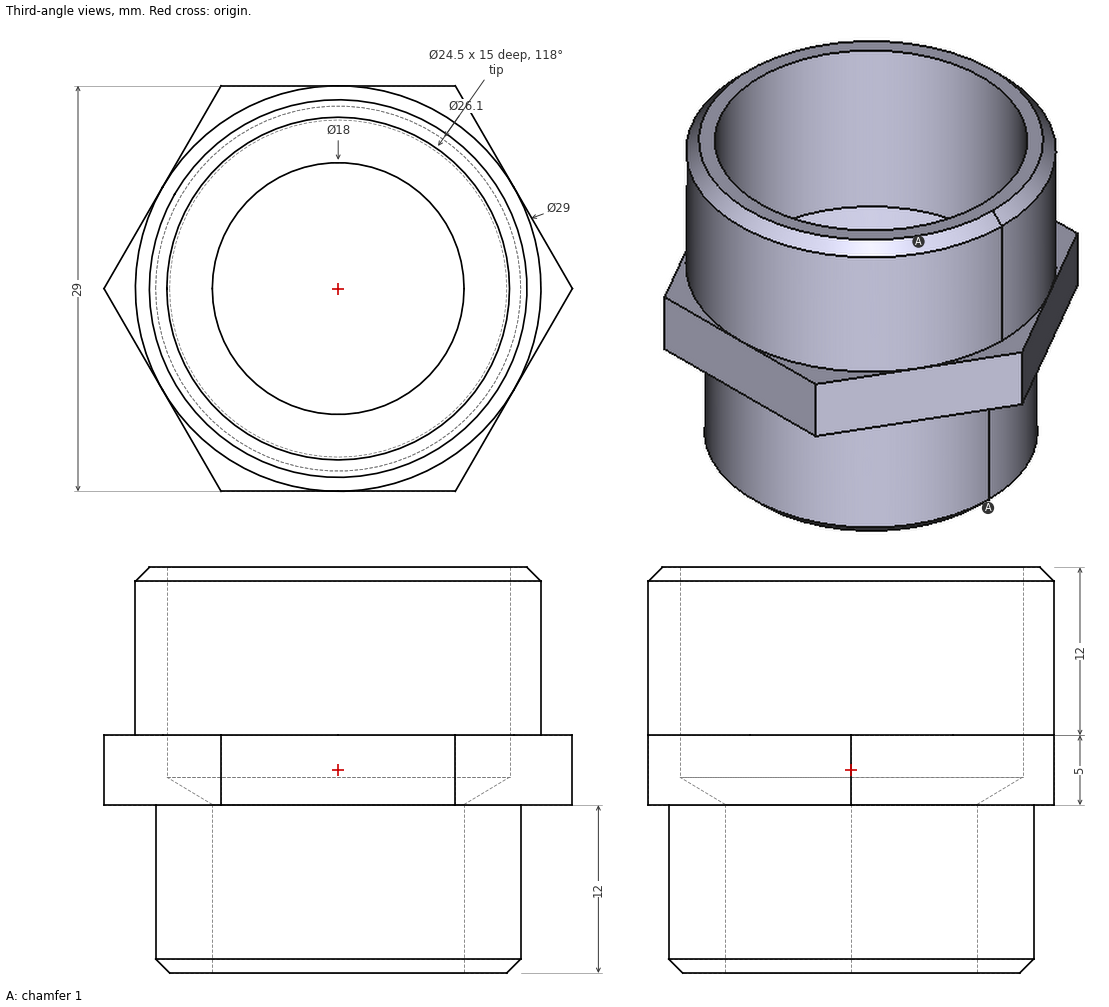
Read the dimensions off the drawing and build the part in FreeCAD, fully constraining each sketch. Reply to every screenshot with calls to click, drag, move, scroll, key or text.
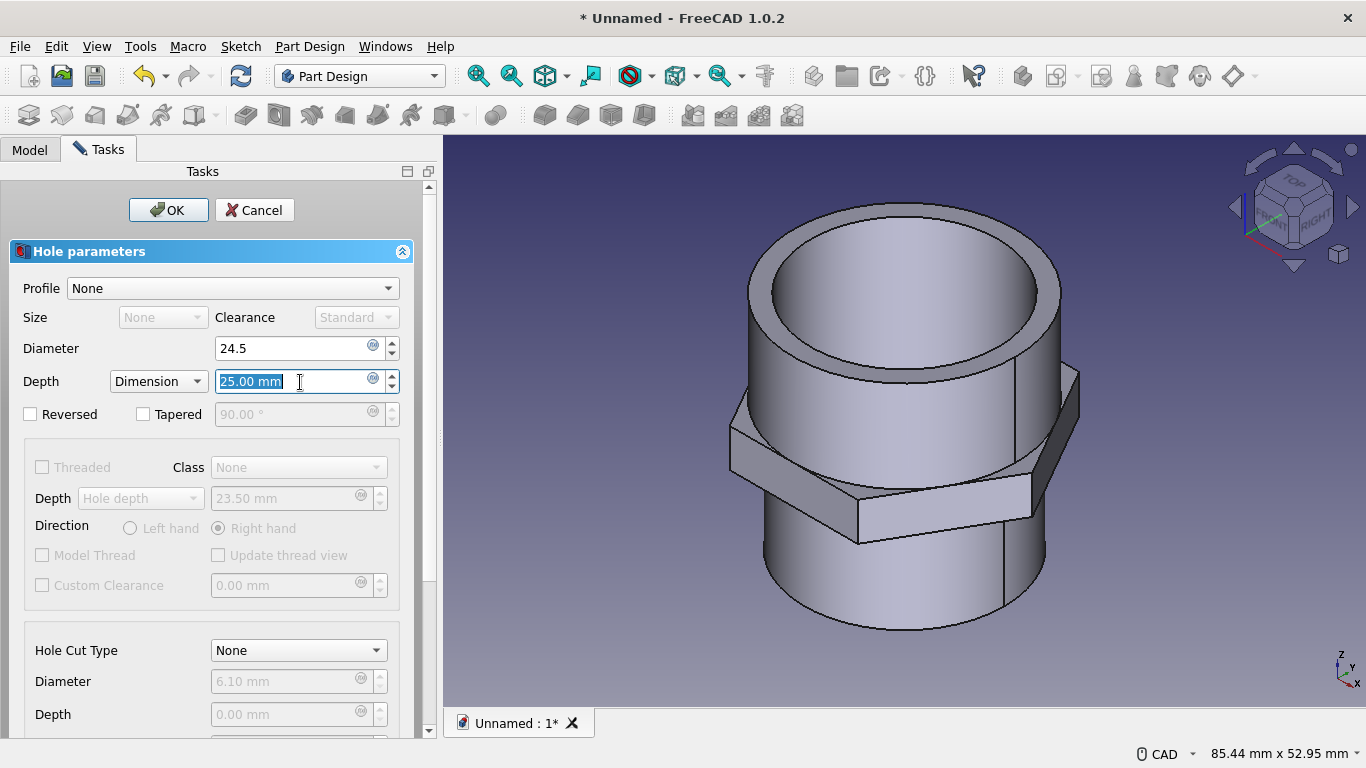
text(15)
key(Tab)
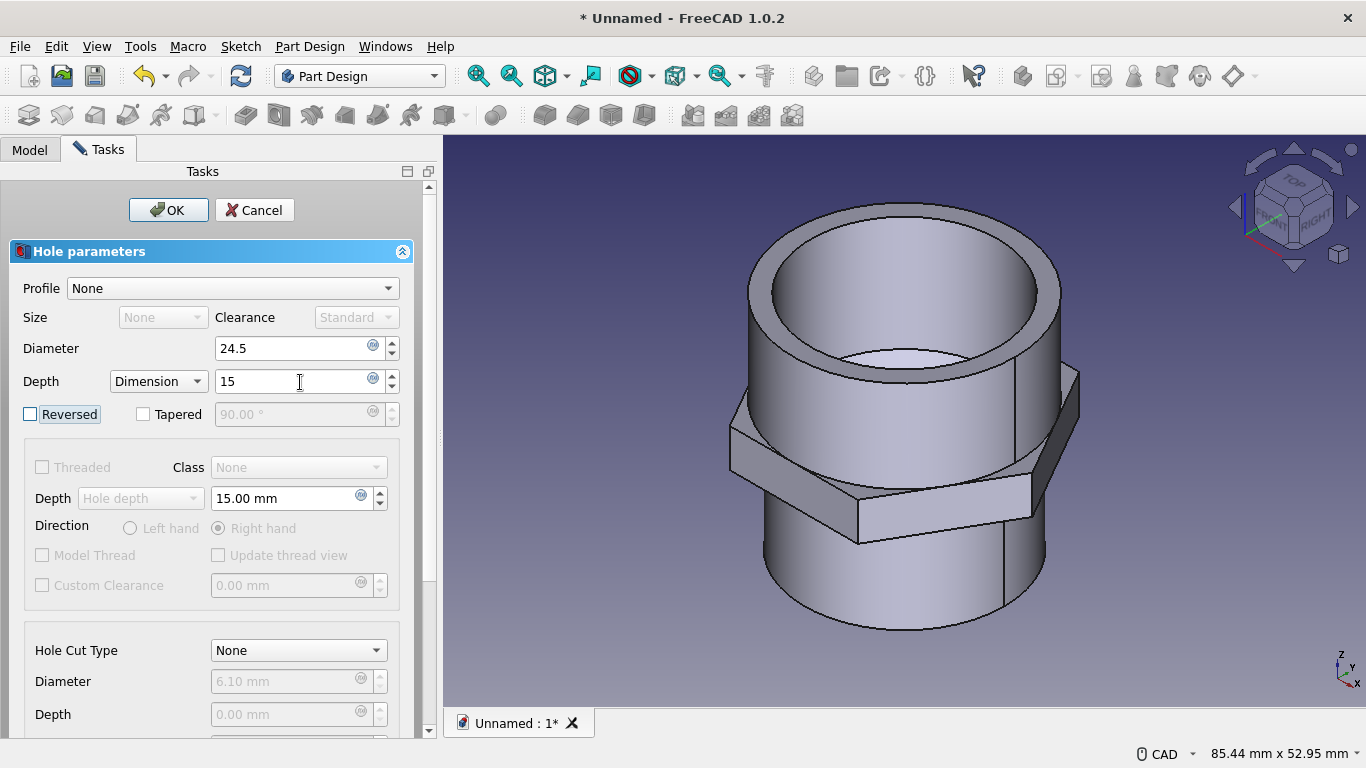
click(169, 210)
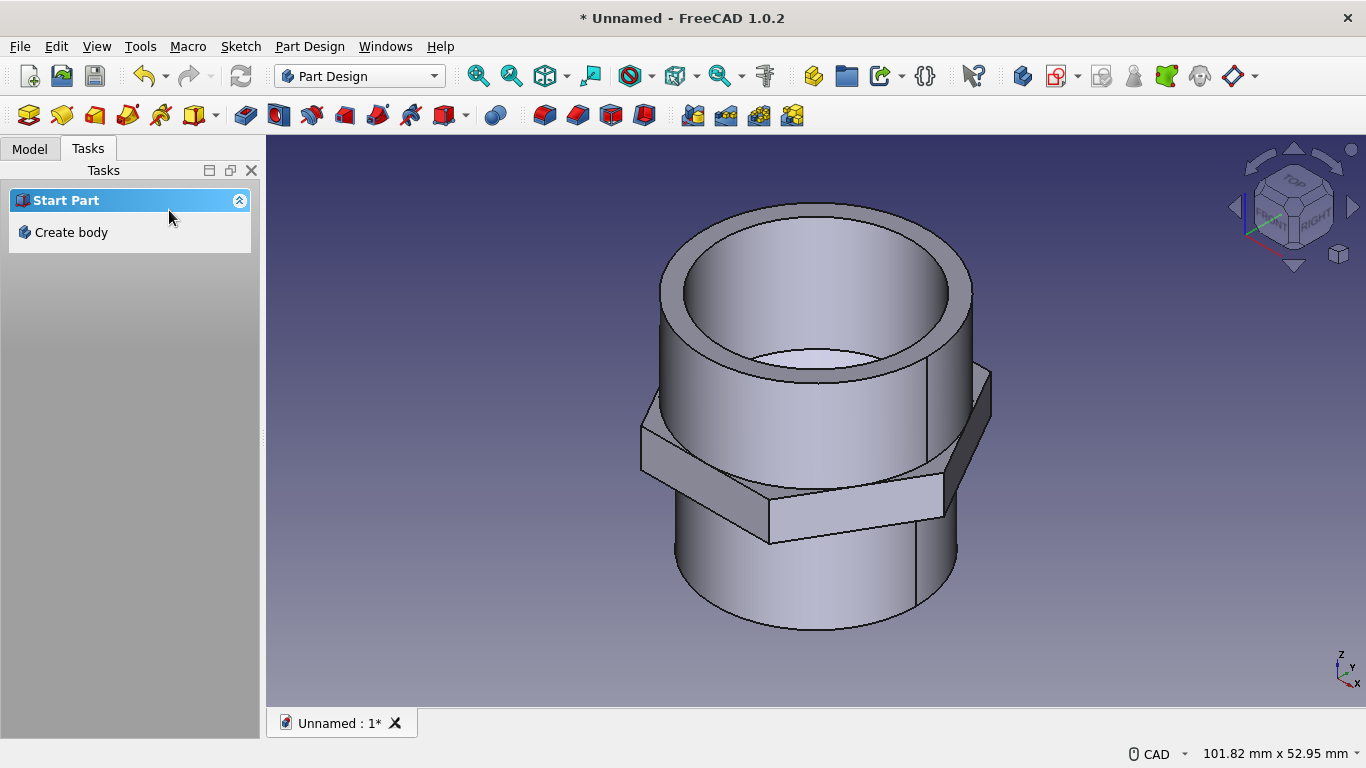
click(676, 333)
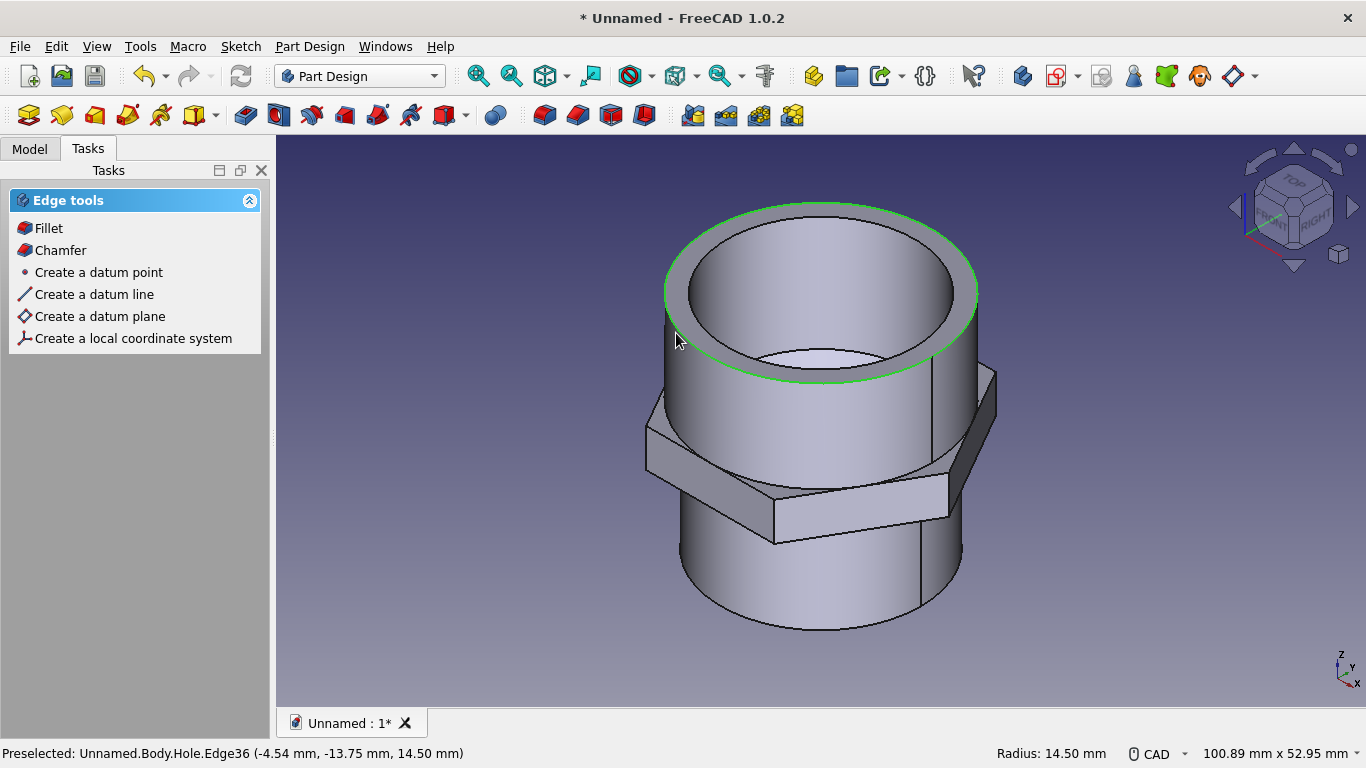
key(2)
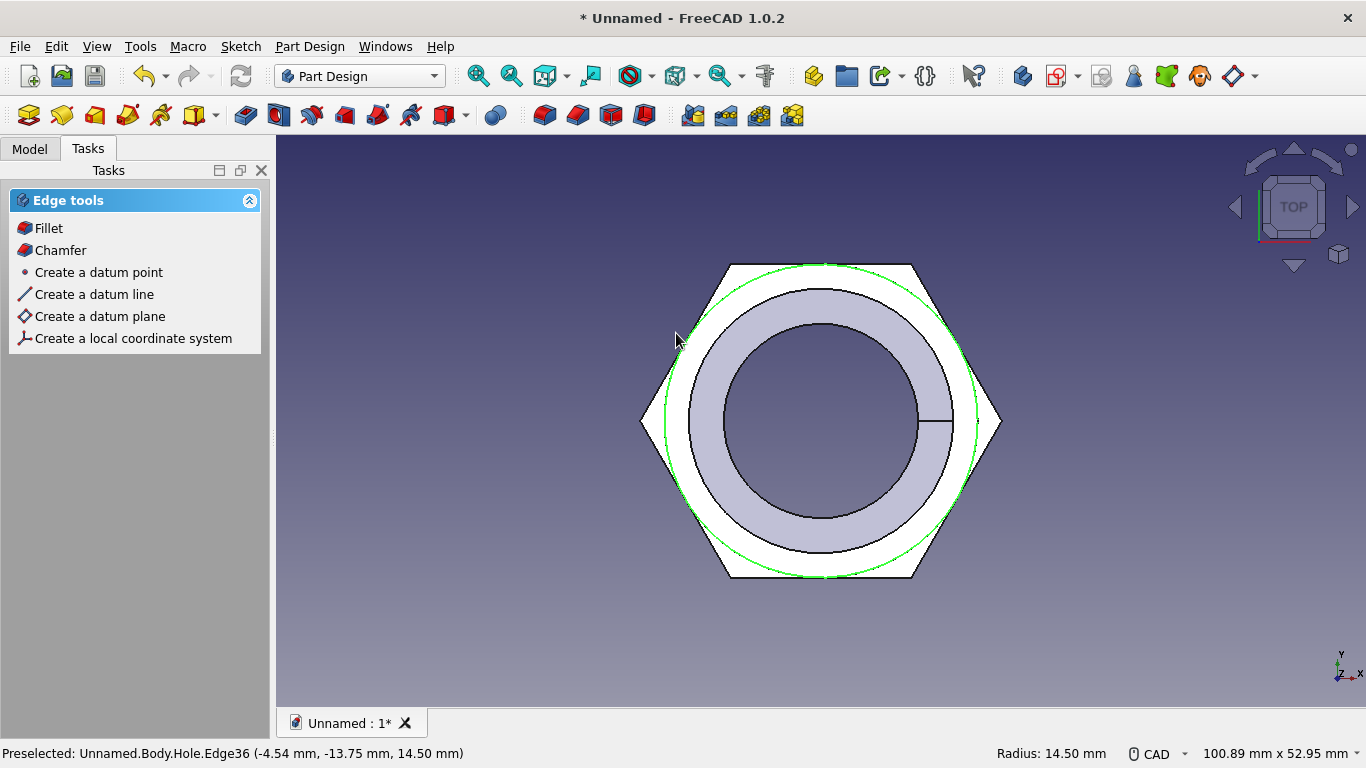
key(0)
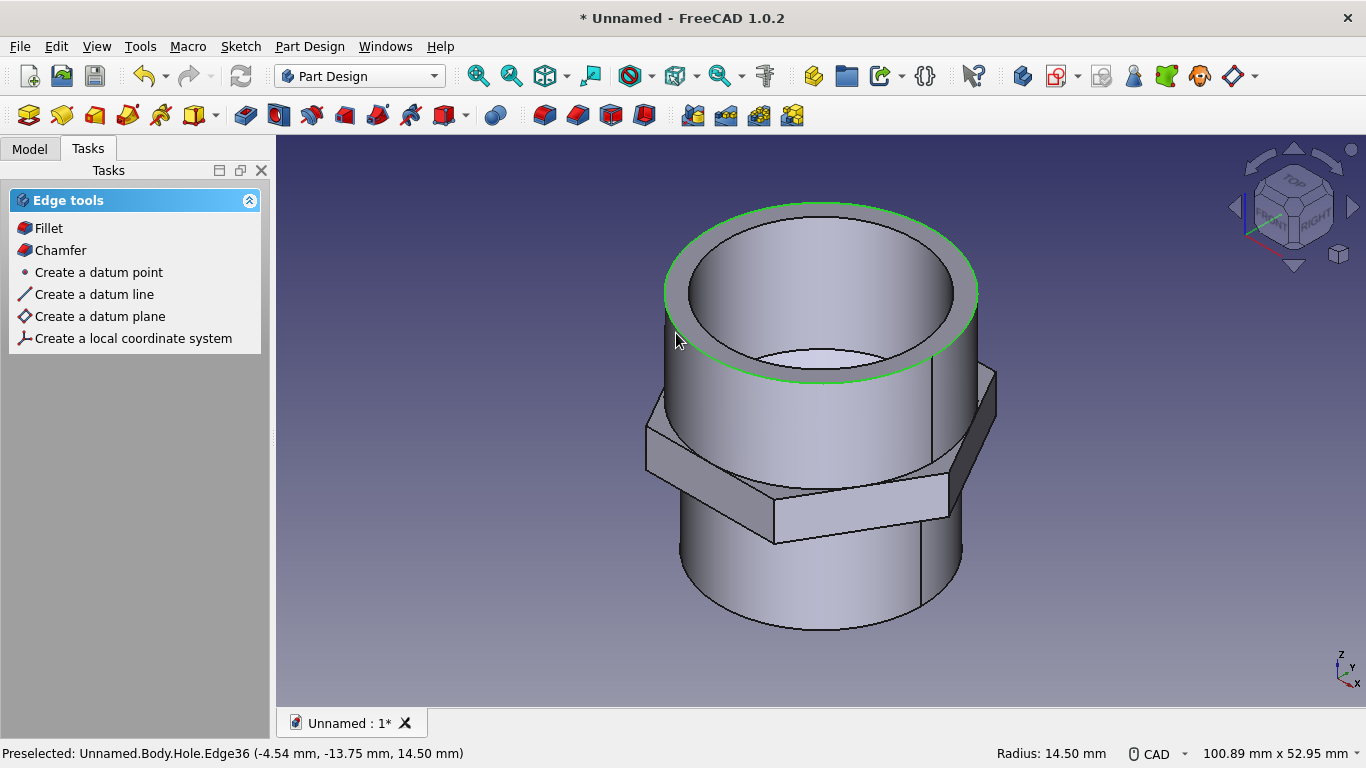
key(1)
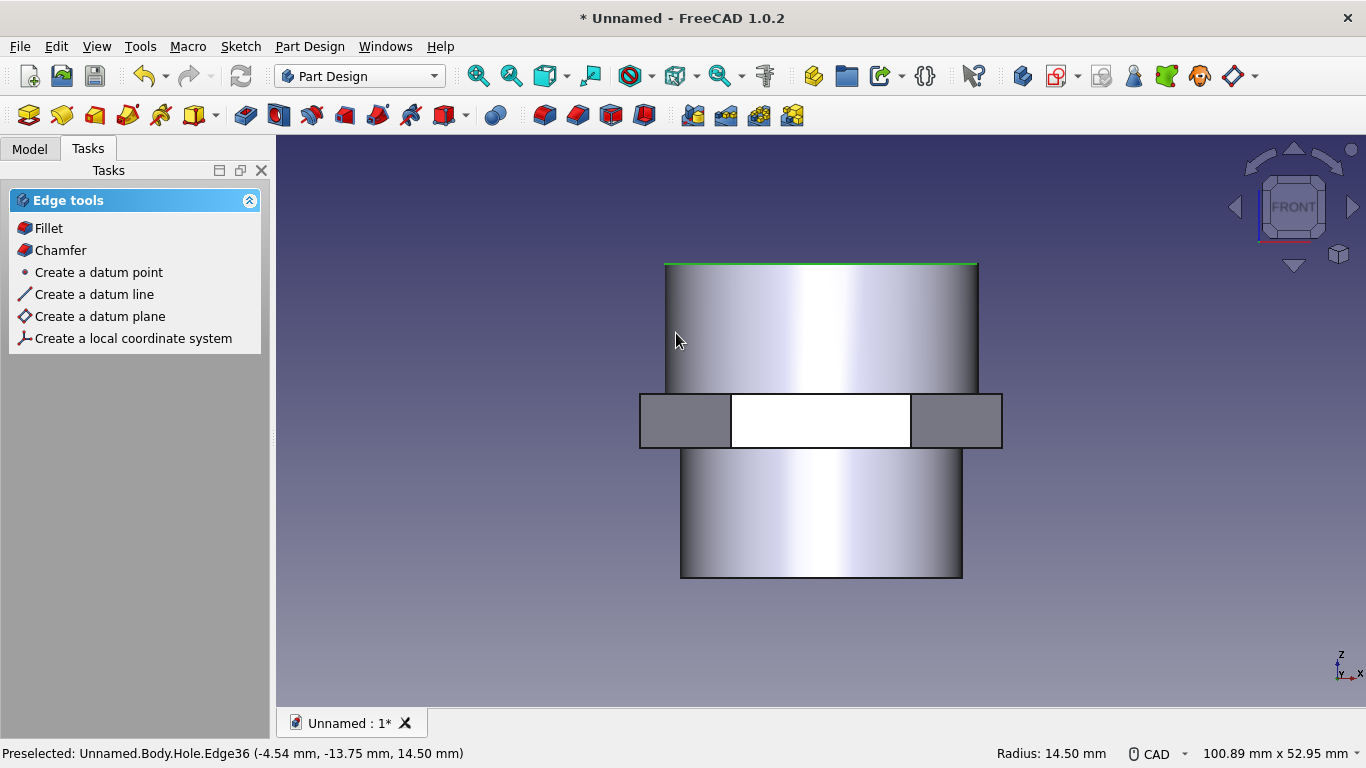
click(707, 577, ctrl)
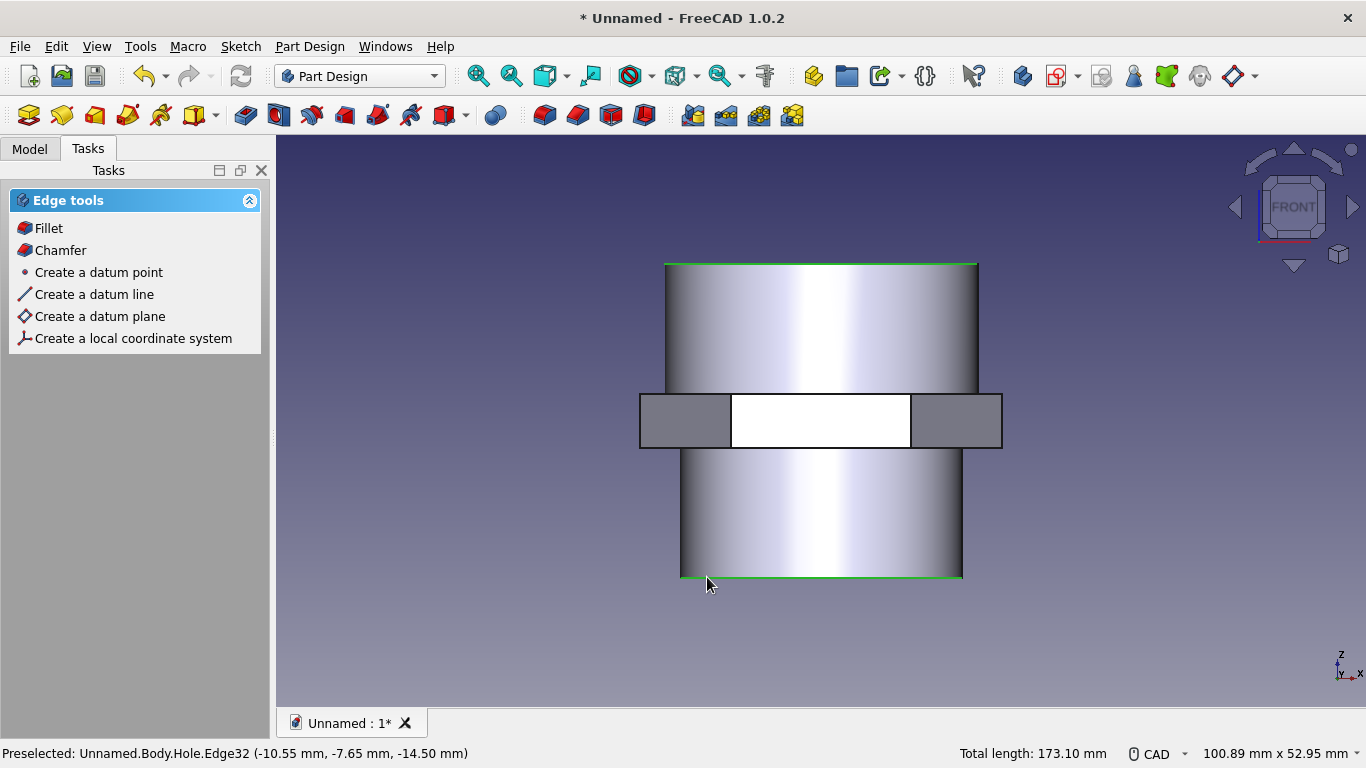
click(578, 116)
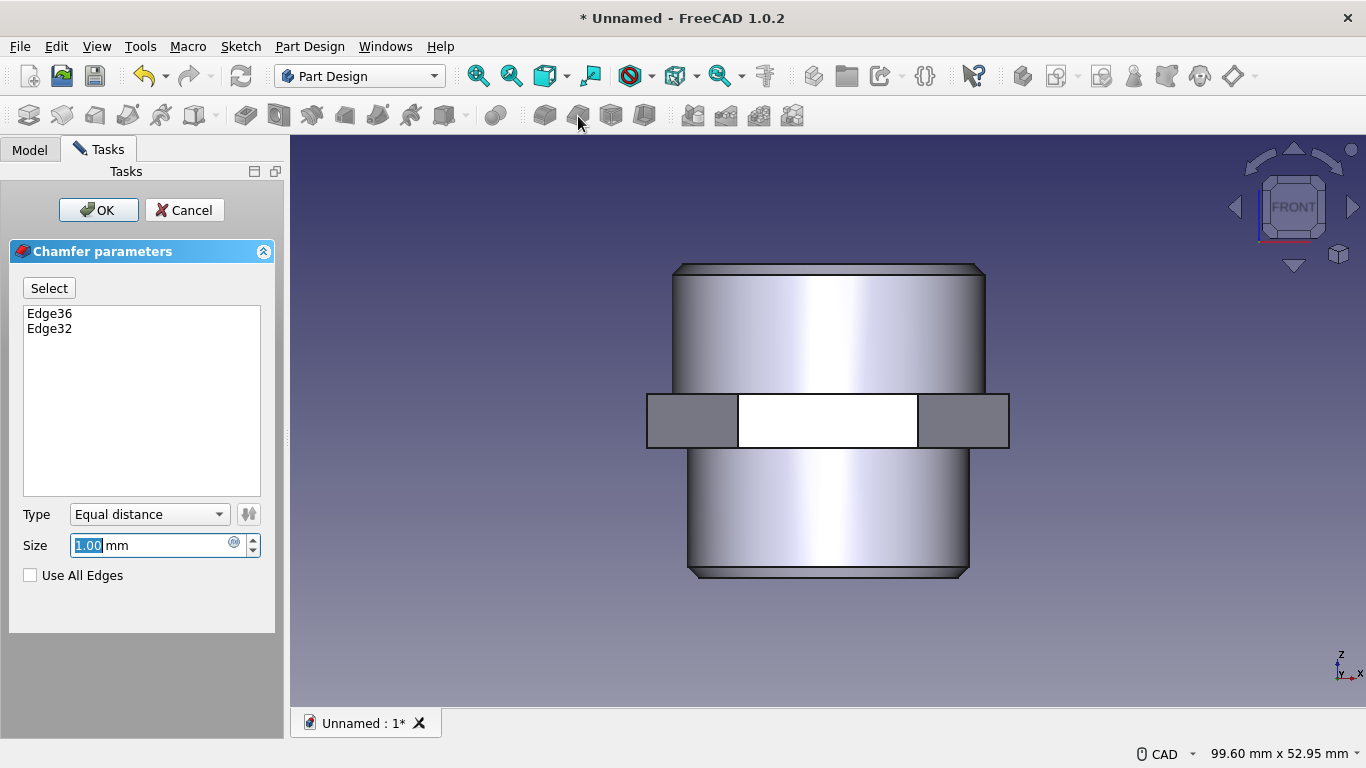
text(1)
key(Tab)